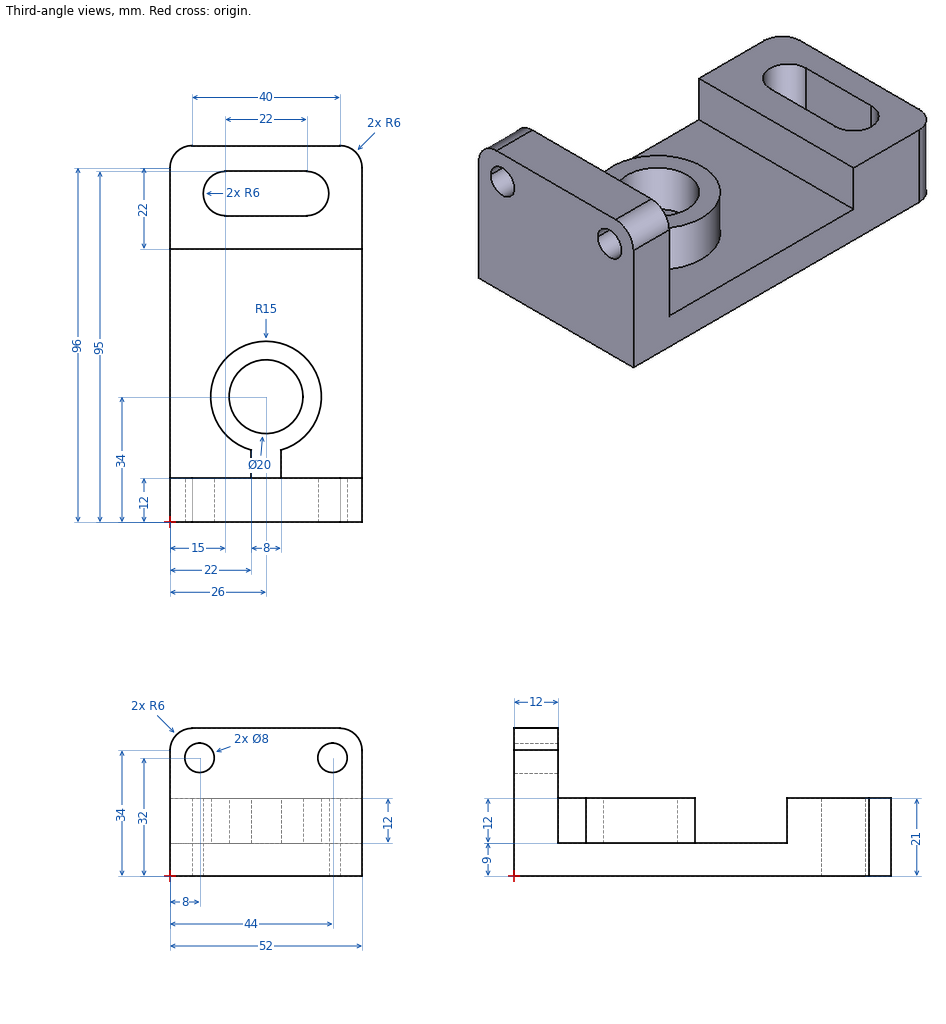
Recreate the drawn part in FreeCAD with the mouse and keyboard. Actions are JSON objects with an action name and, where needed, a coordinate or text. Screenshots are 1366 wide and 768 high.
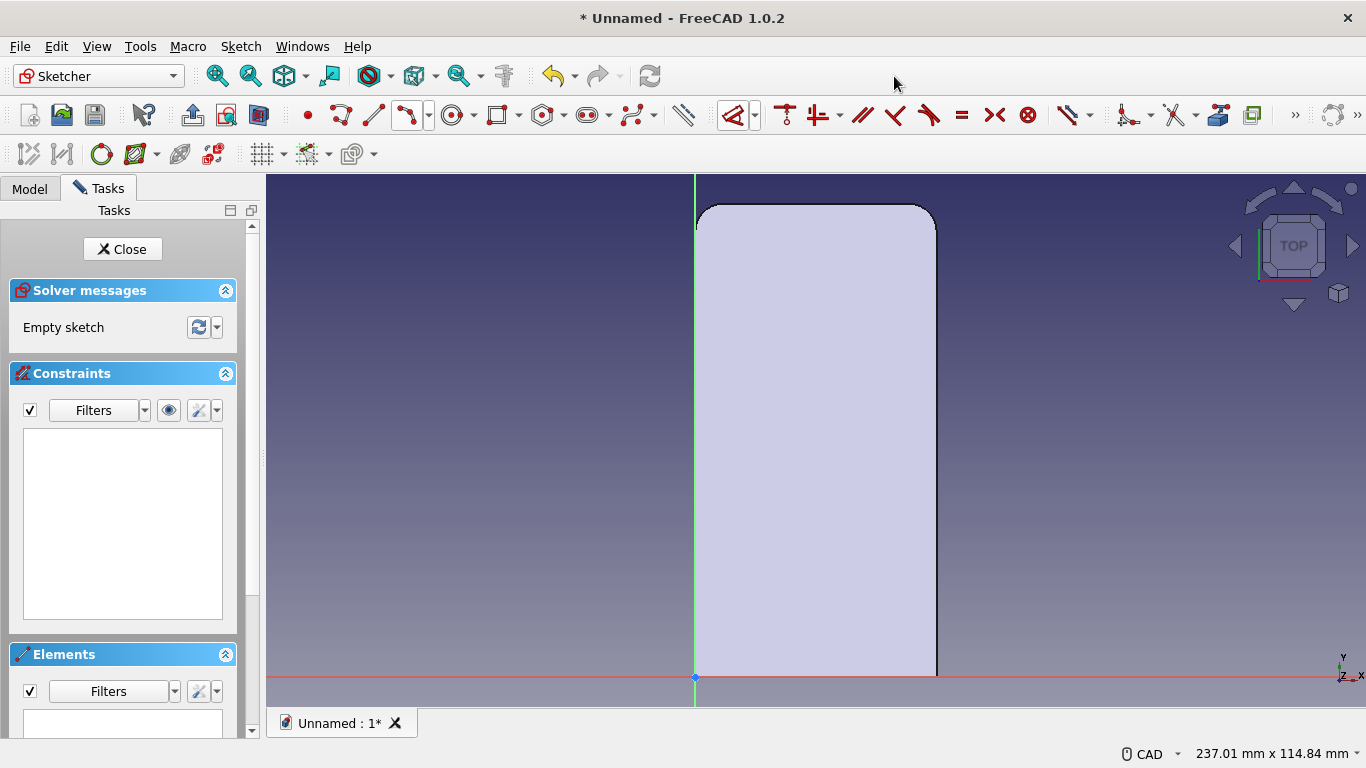
{"action": "scroll", "coordinate": [608, 440], "scroll_direction": "down", "scroll_amount": 2}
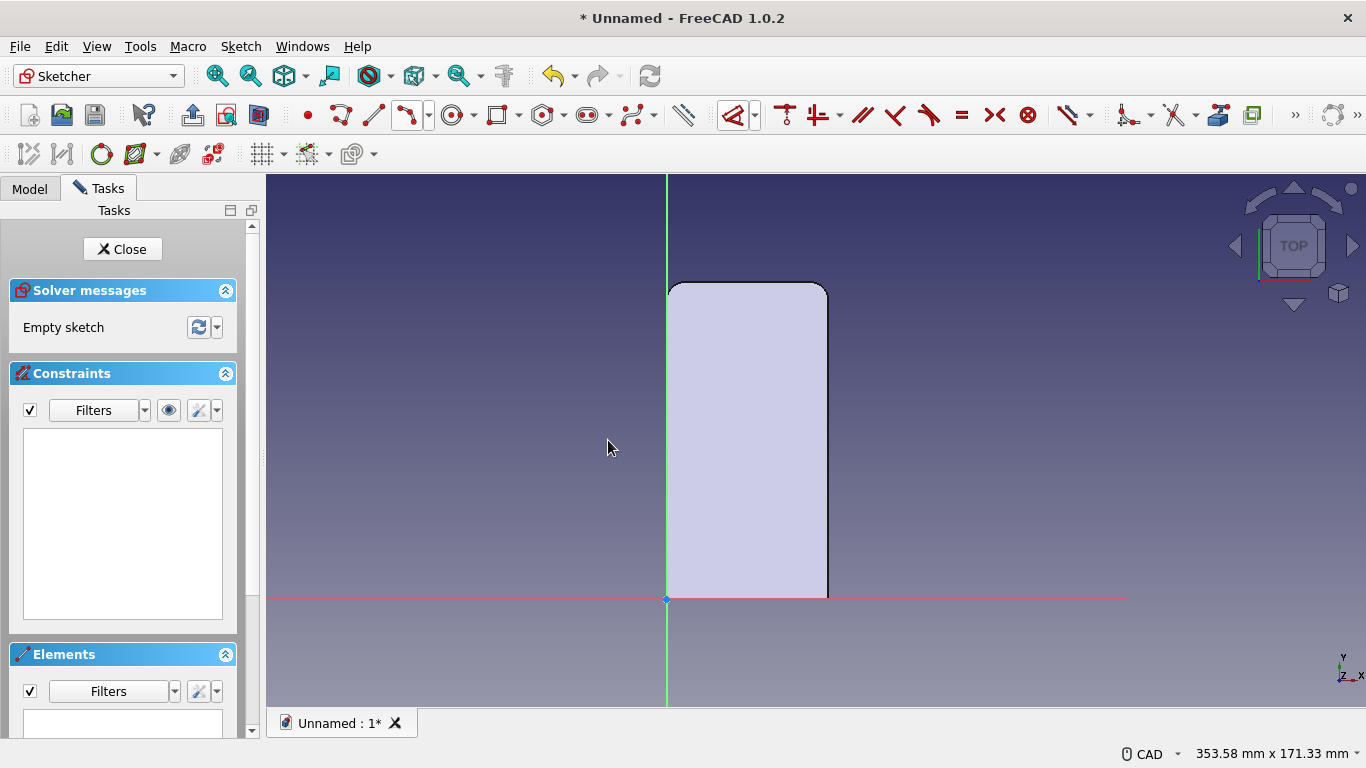
{"action": "left_click", "coordinate": [374, 116]}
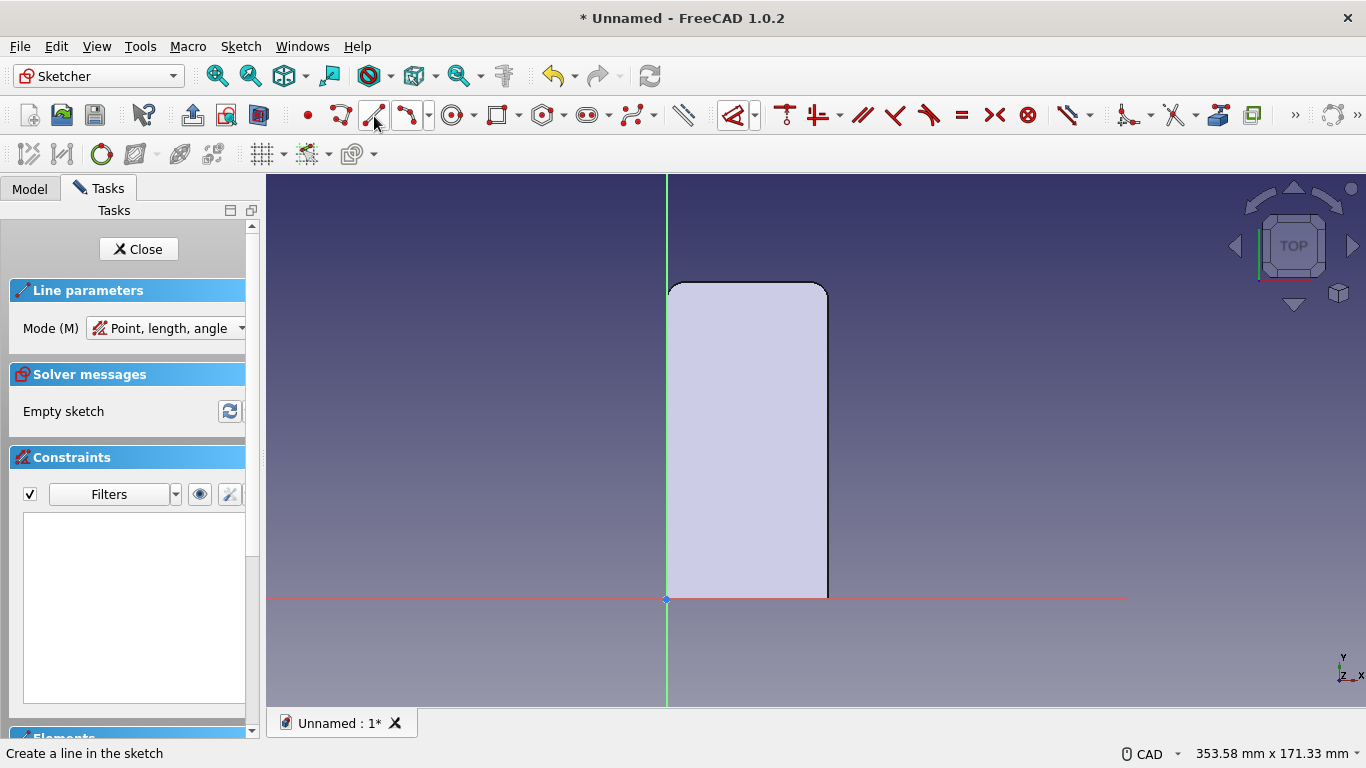
{"action": "left_click", "coordinate": [810, 282]}
{"action": "left_click", "coordinate": [685, 282]}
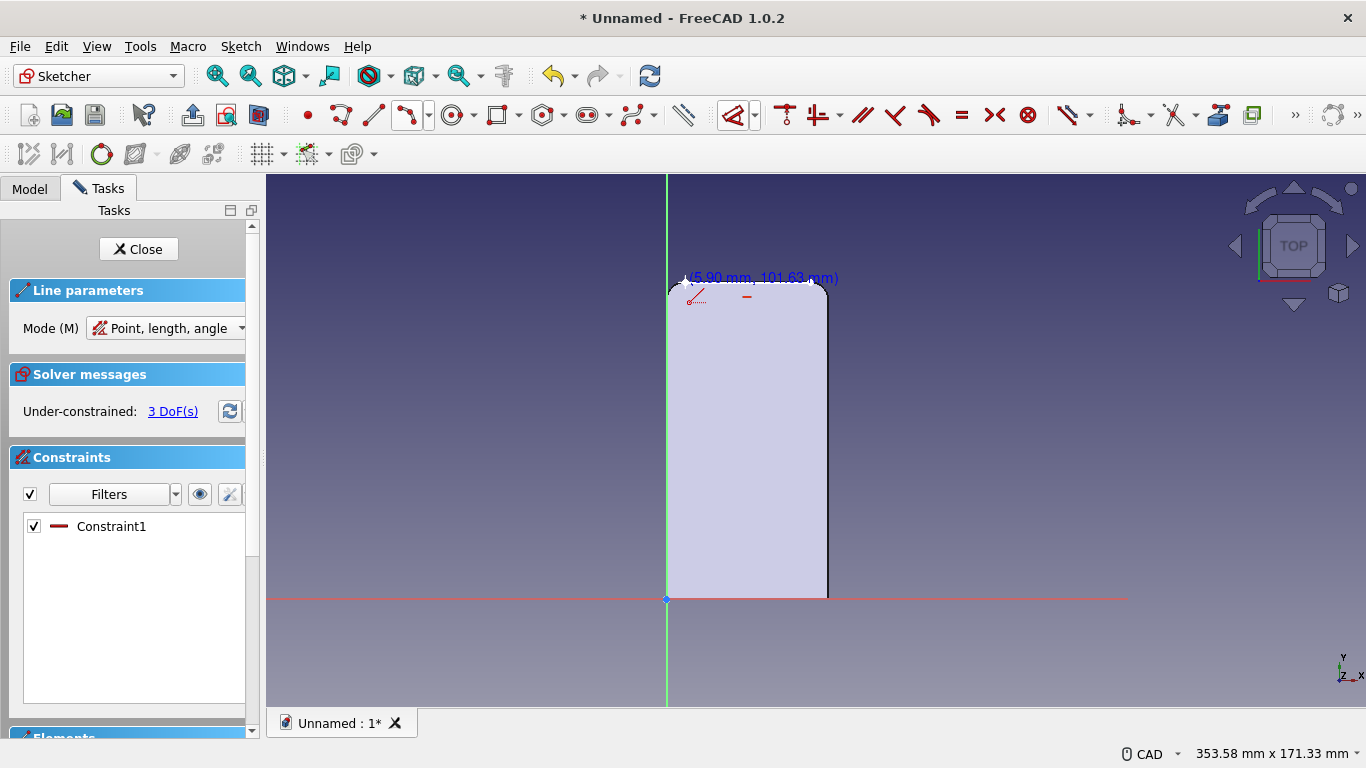
{"action": "left_click", "coordinate": [341, 116]}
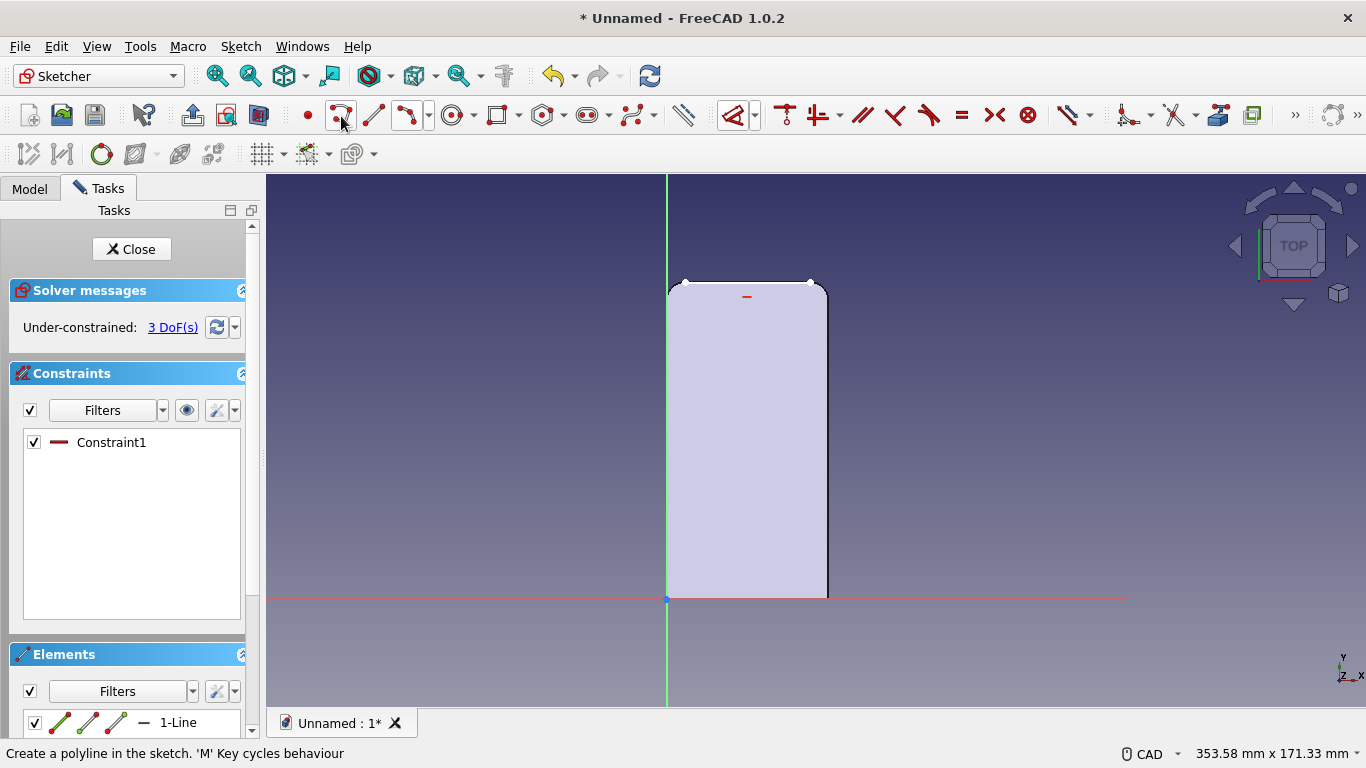
{"action": "left_click", "coordinate": [667, 301]}
{"action": "left_click", "coordinate": [676, 369]}
{"action": "left_click", "coordinate": [828, 369]}
{"action": "left_click", "coordinate": [828, 301]}
{"action": "right_click", "coordinate": [828, 301]}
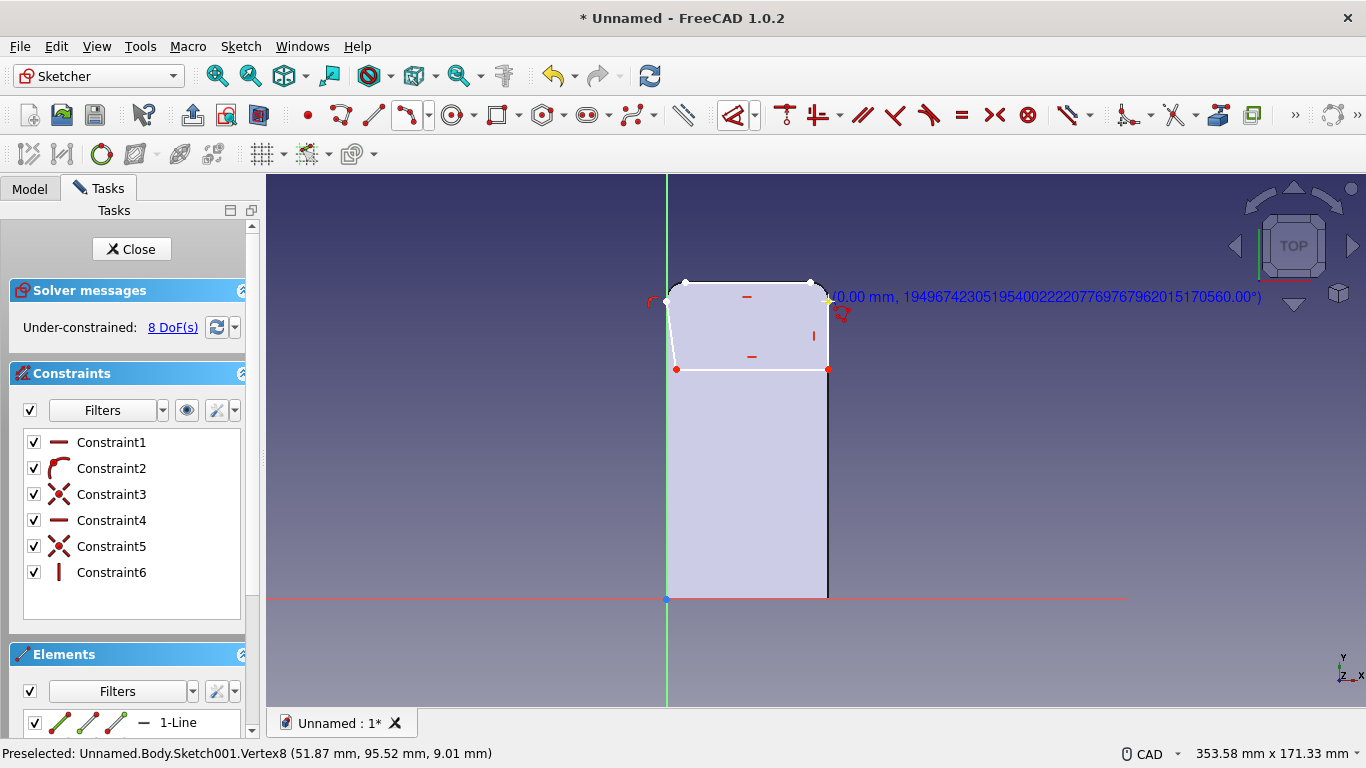
{"action": "left_click", "coordinate": [406, 116]}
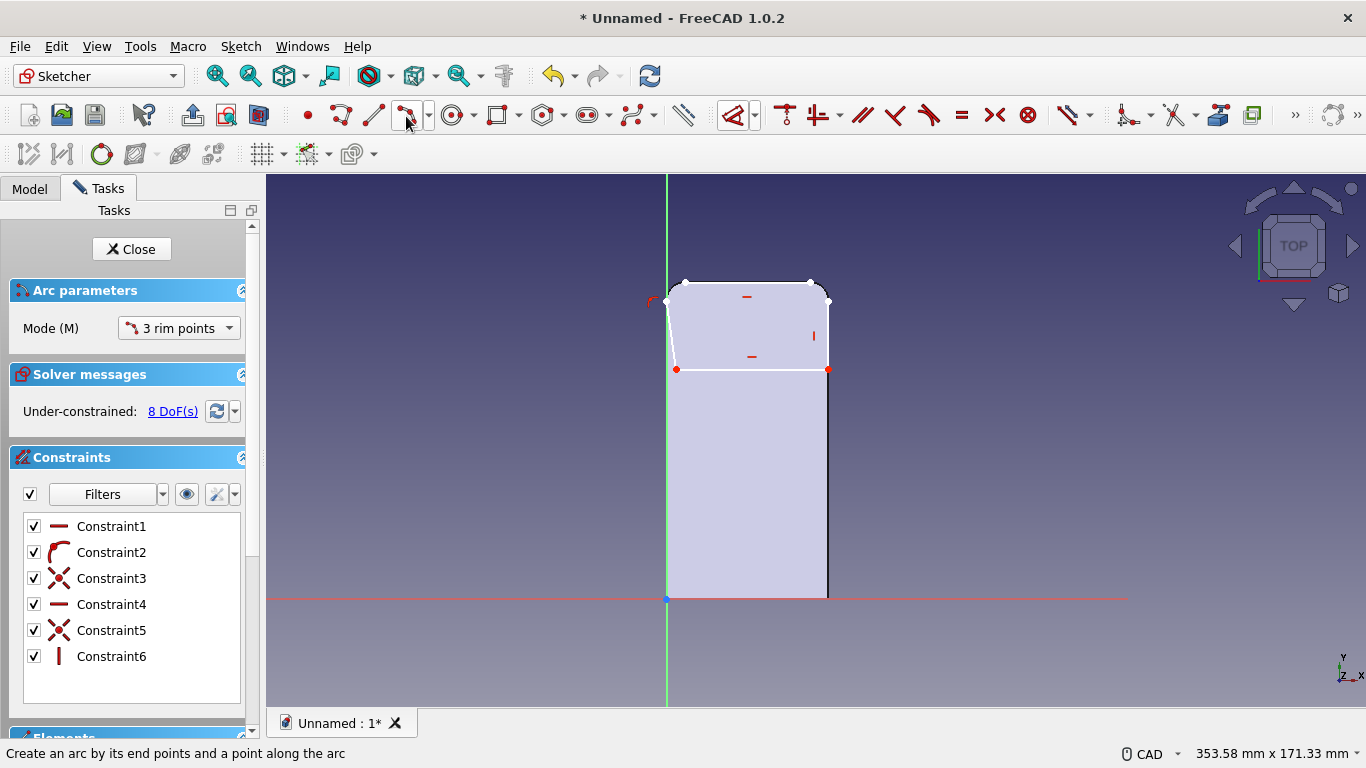
{"action": "left_click", "coordinate": [685, 283]}
{"action": "left_click", "coordinate": [667, 302]}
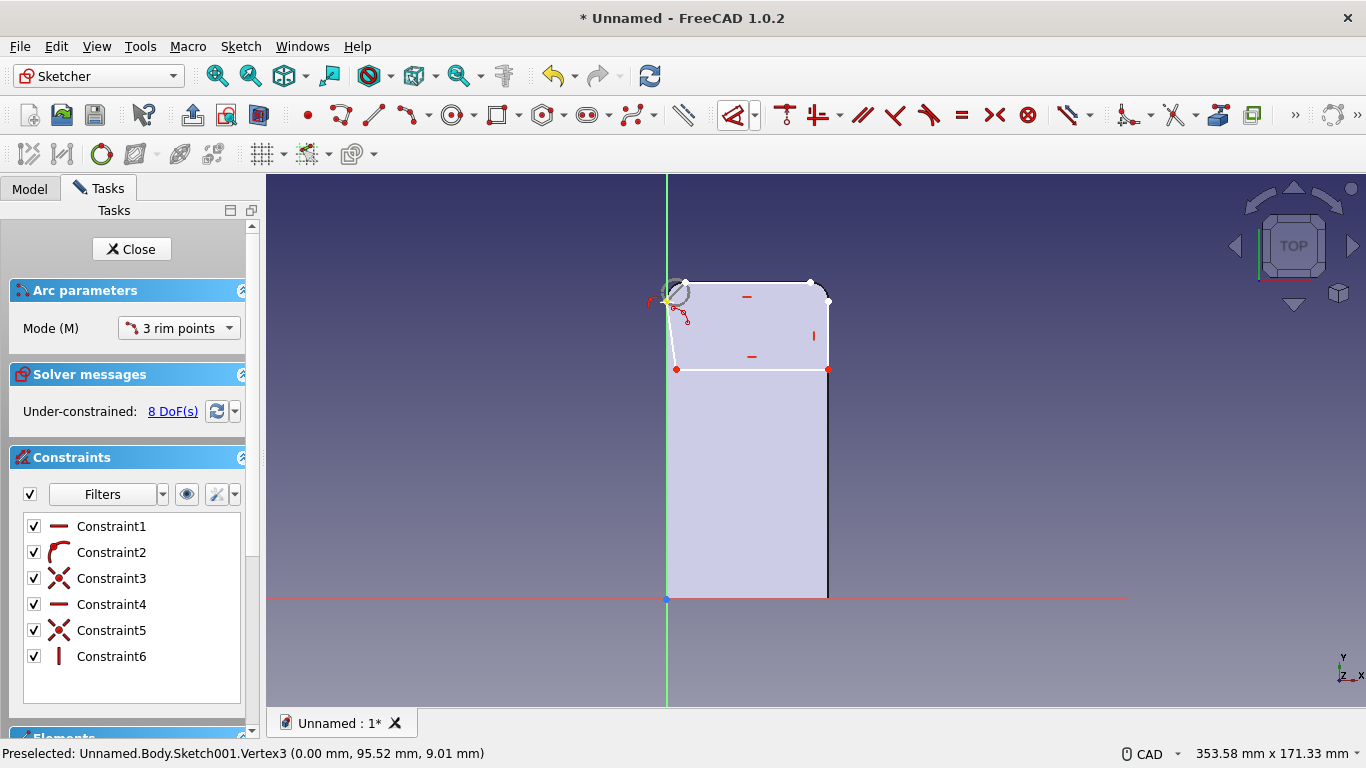
{"action": "scroll", "coordinate": [672, 287], "scroll_direction": "up", "scroll_amount": 6}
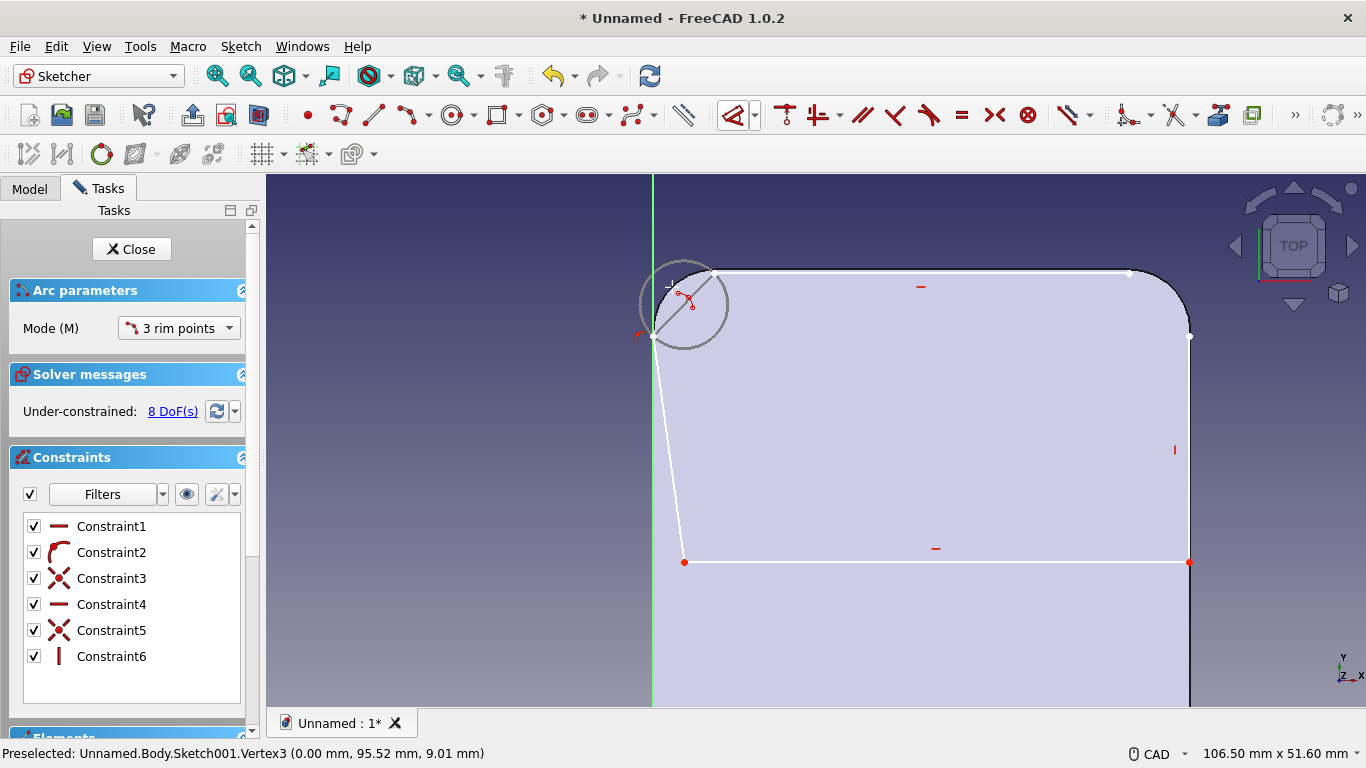
{"action": "left_click", "coordinate": [672, 288]}